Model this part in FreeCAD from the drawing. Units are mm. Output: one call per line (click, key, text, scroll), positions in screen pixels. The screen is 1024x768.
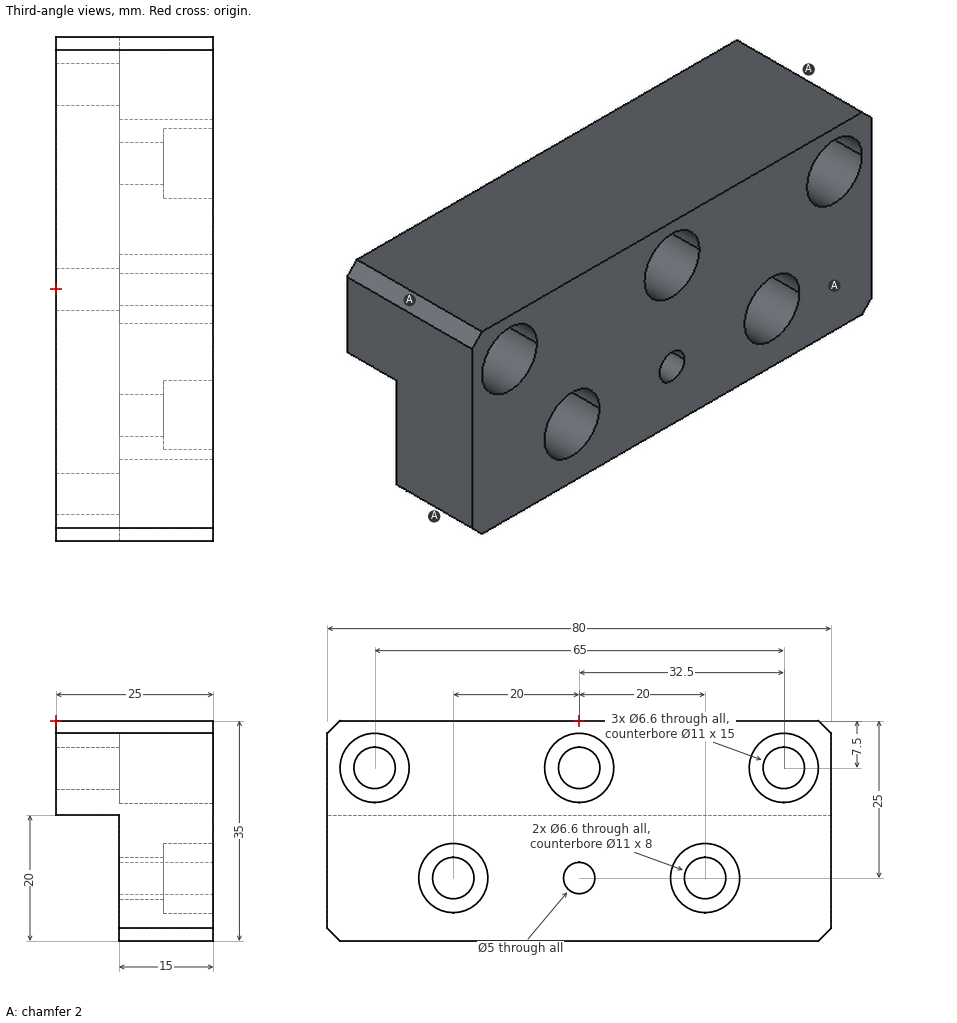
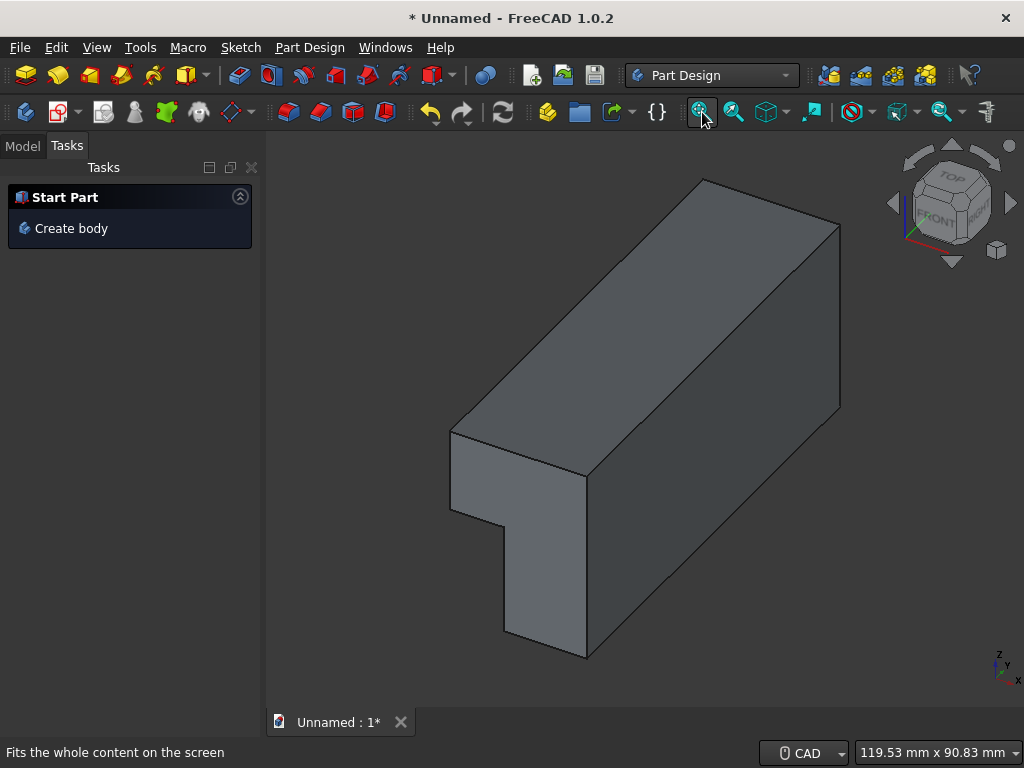
click(518, 453)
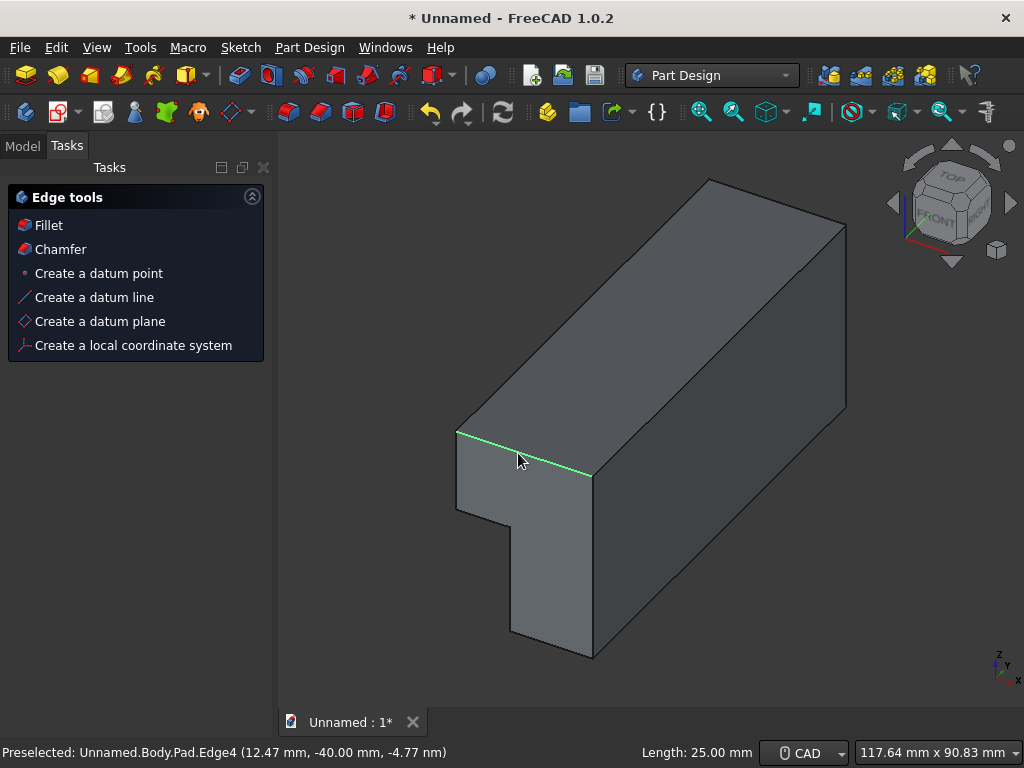
key(0)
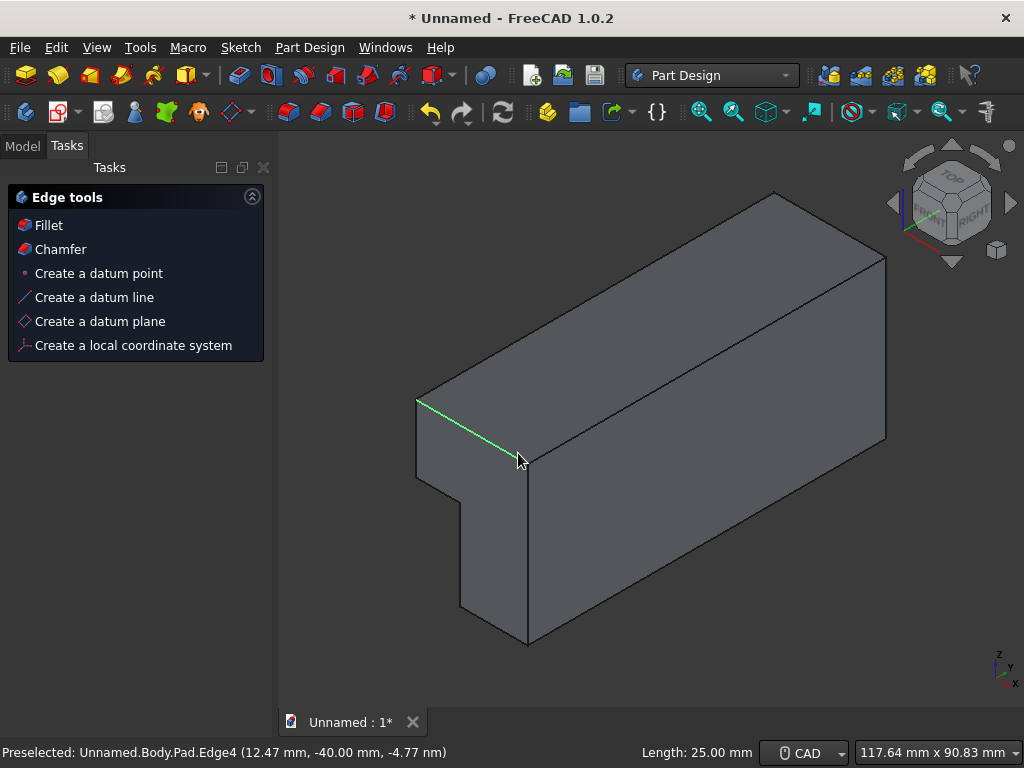
key(2)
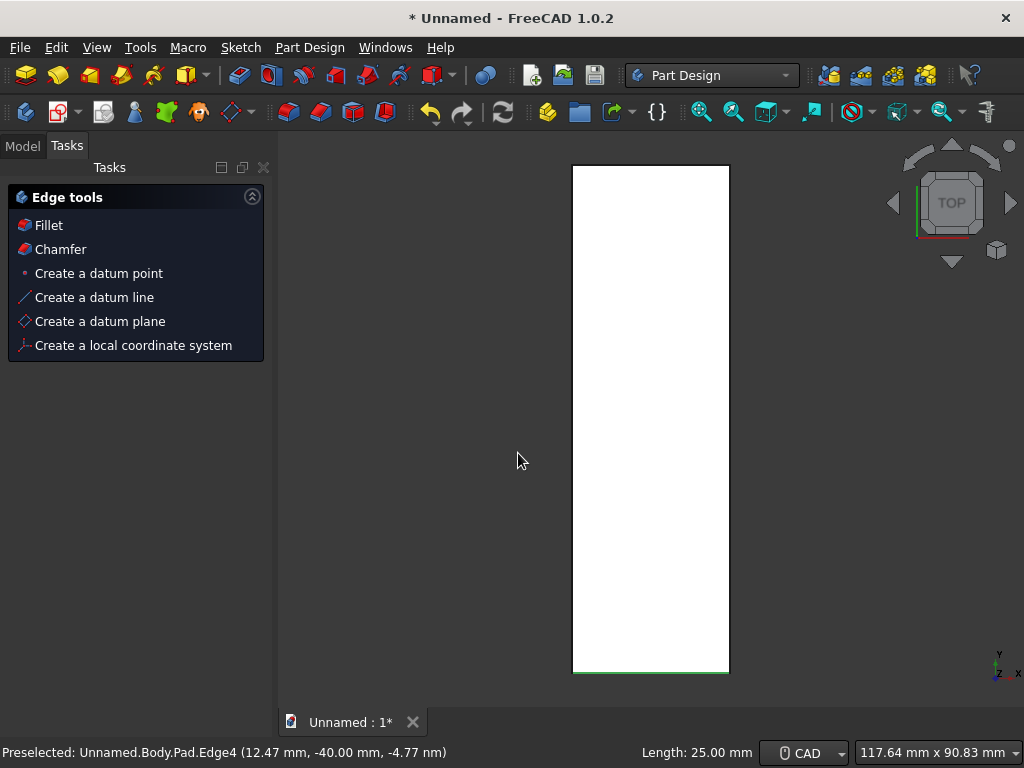
click(651, 164, ctrl)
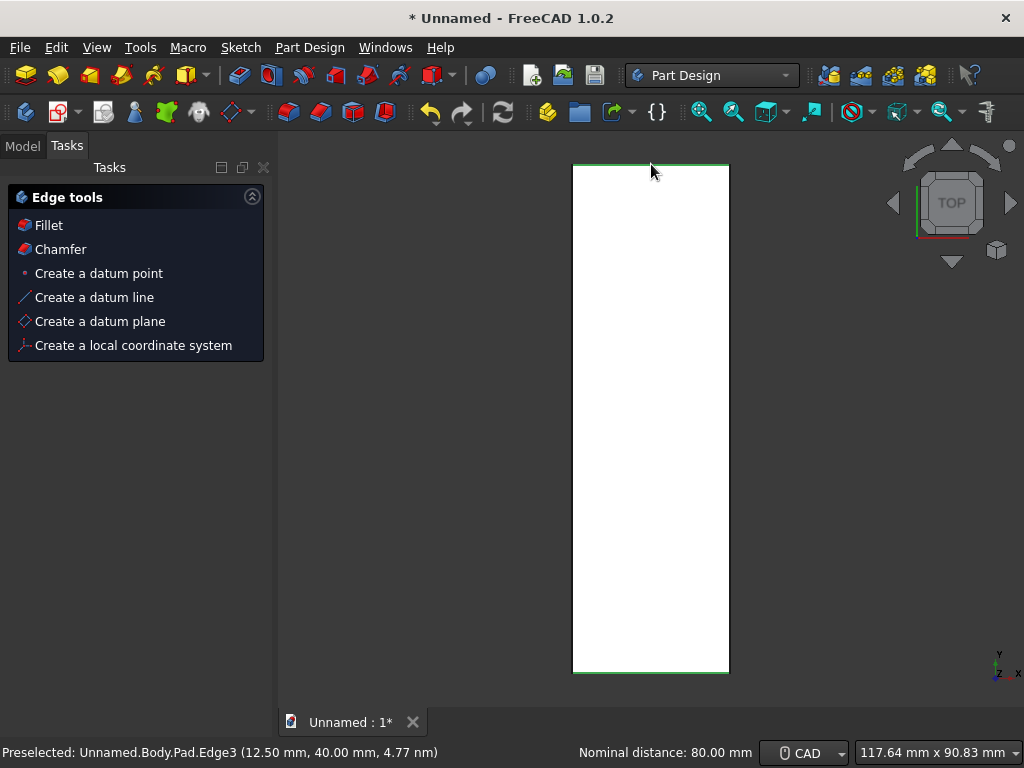
key(1)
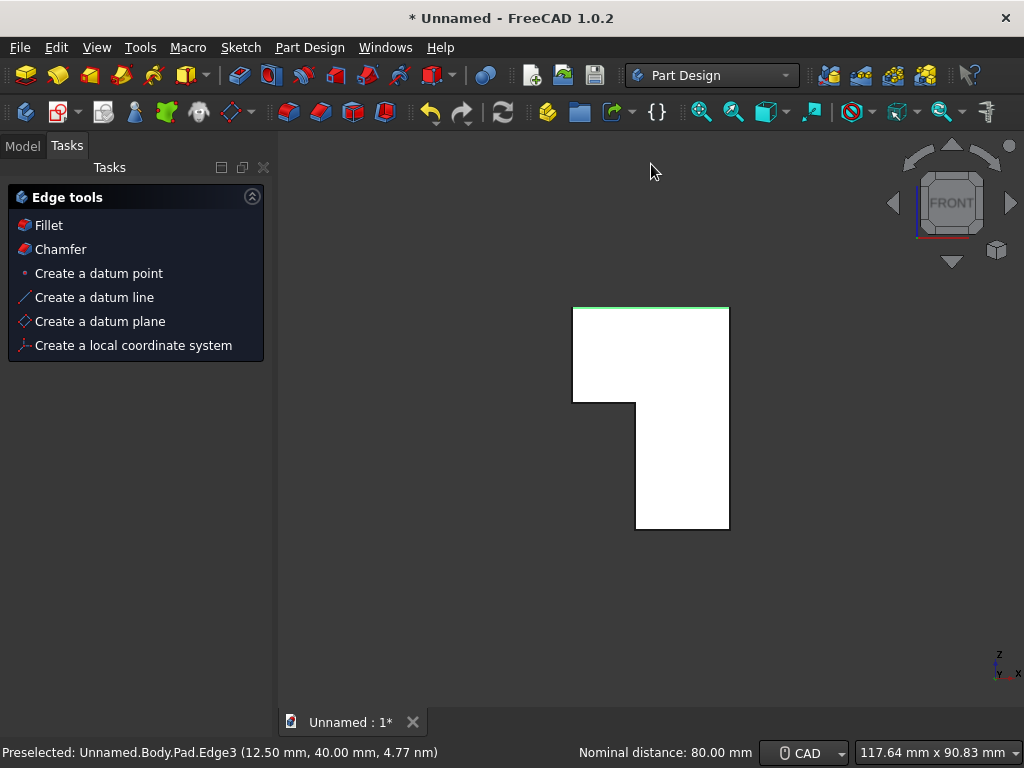
key(v)
key(f)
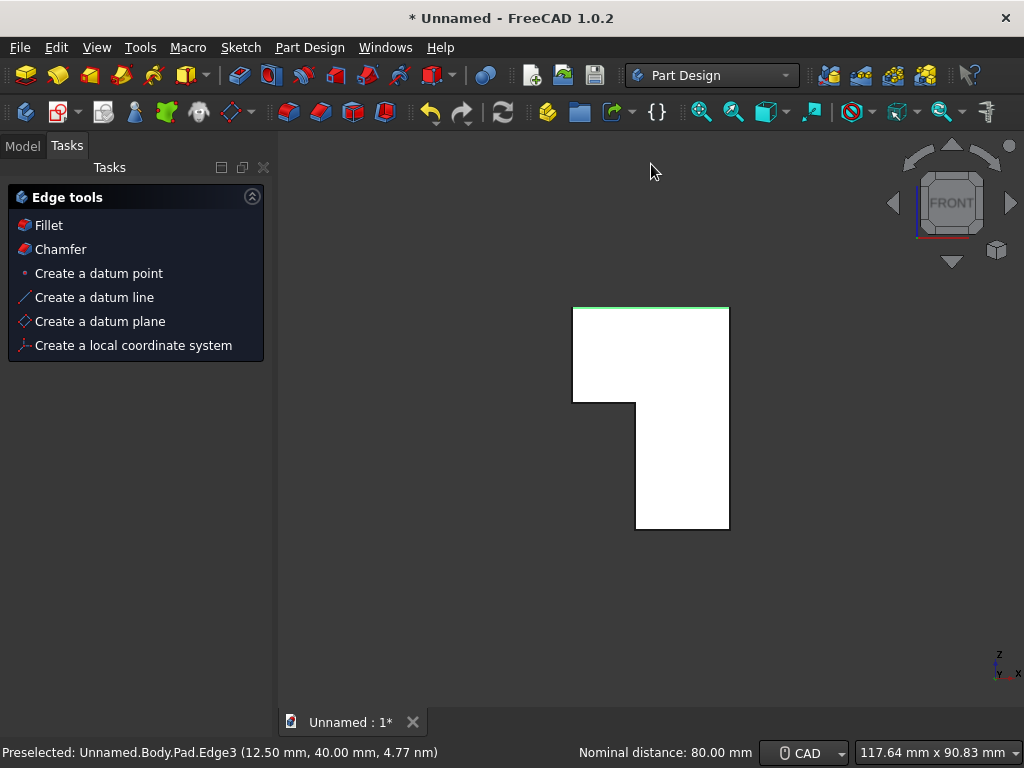
key(3)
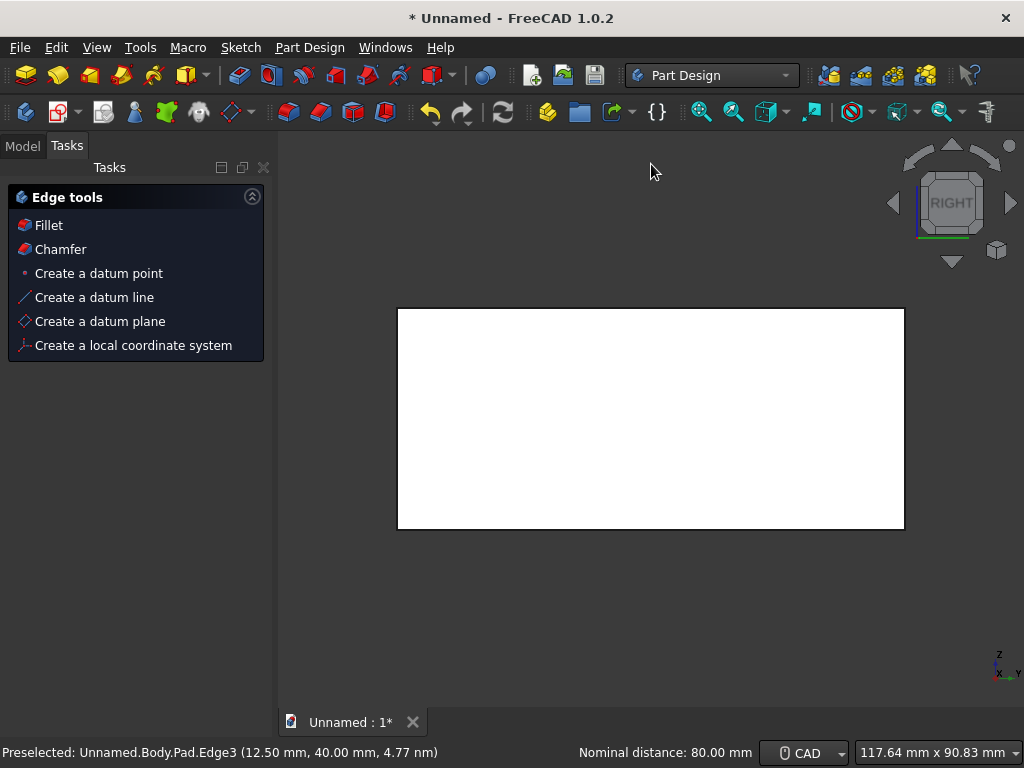
key(5)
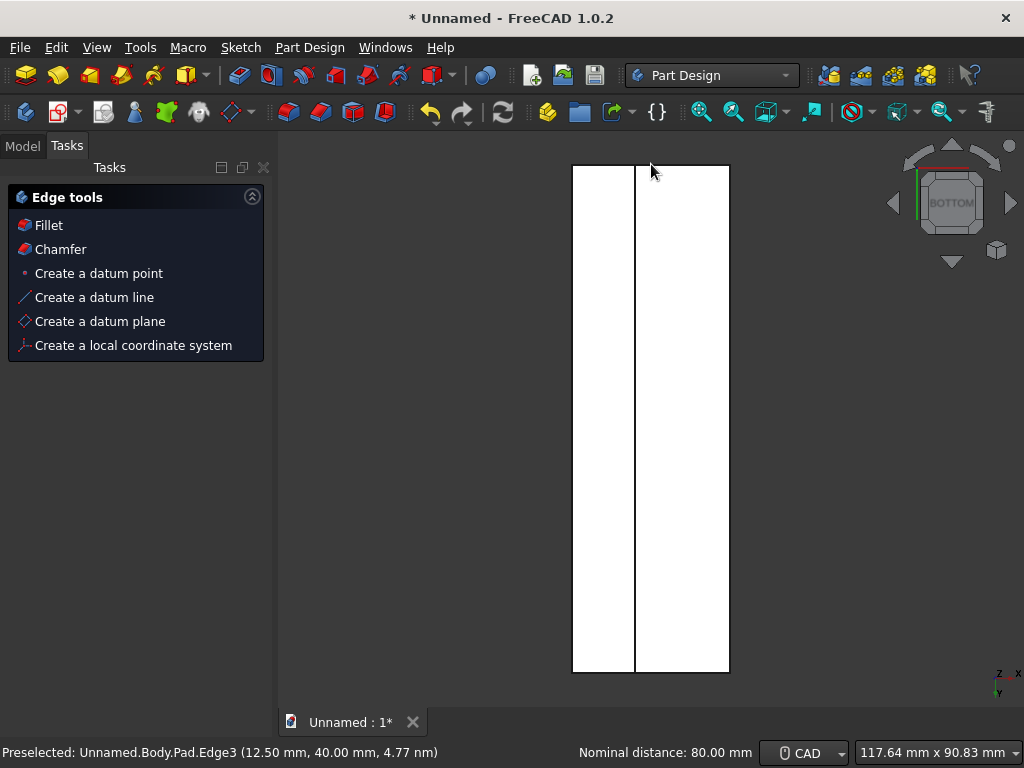
click(683, 164, ctrl)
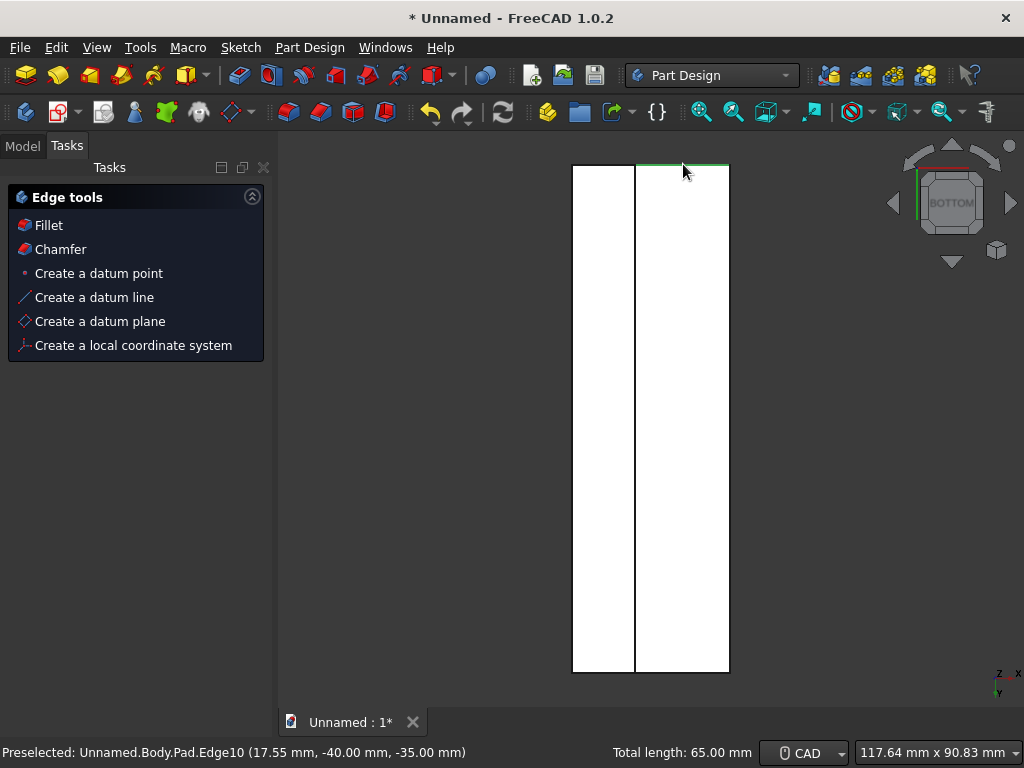
key(4)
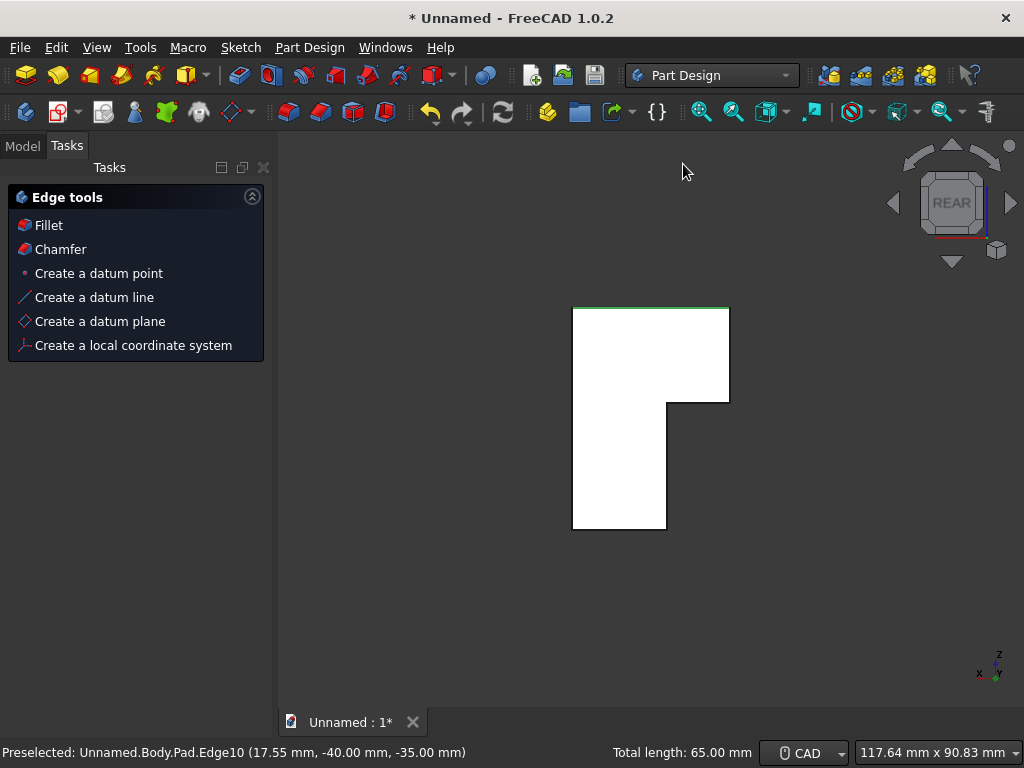
click(702, 112)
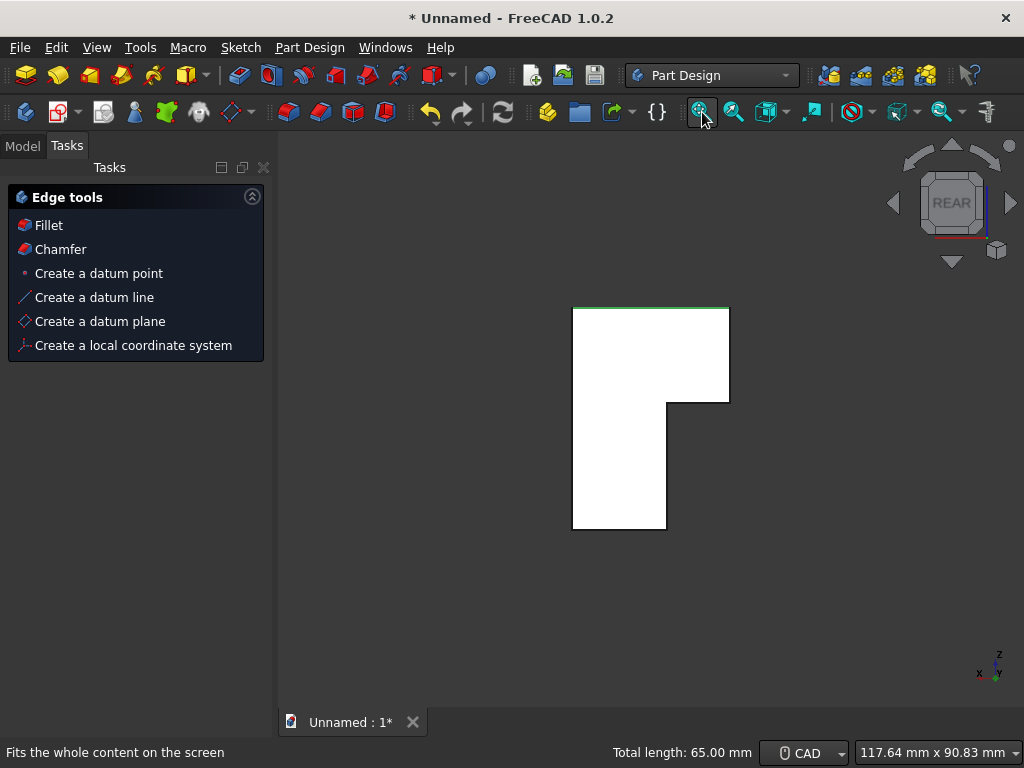
click(619, 529, ctrl)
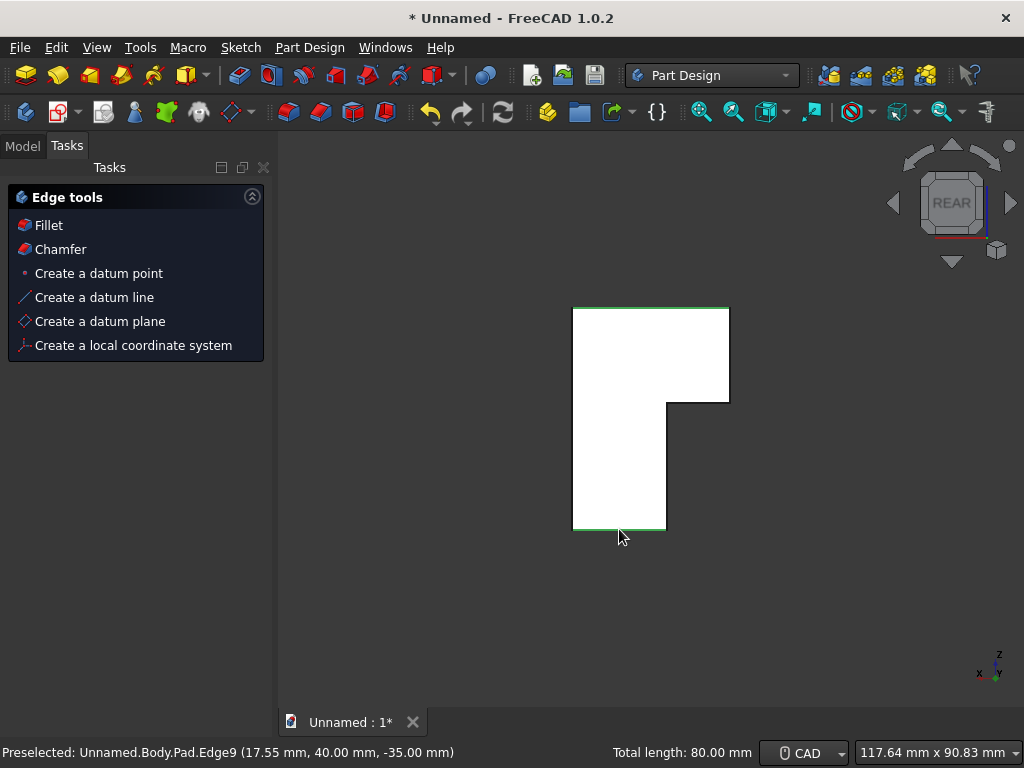
click(322, 112)